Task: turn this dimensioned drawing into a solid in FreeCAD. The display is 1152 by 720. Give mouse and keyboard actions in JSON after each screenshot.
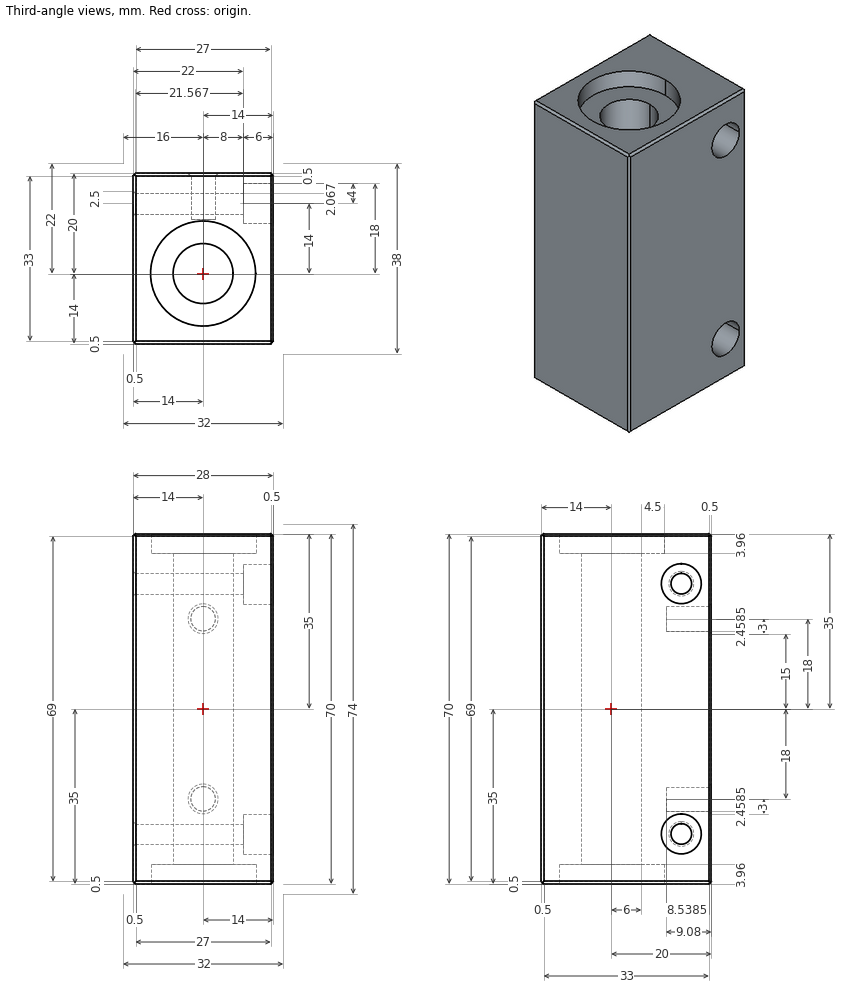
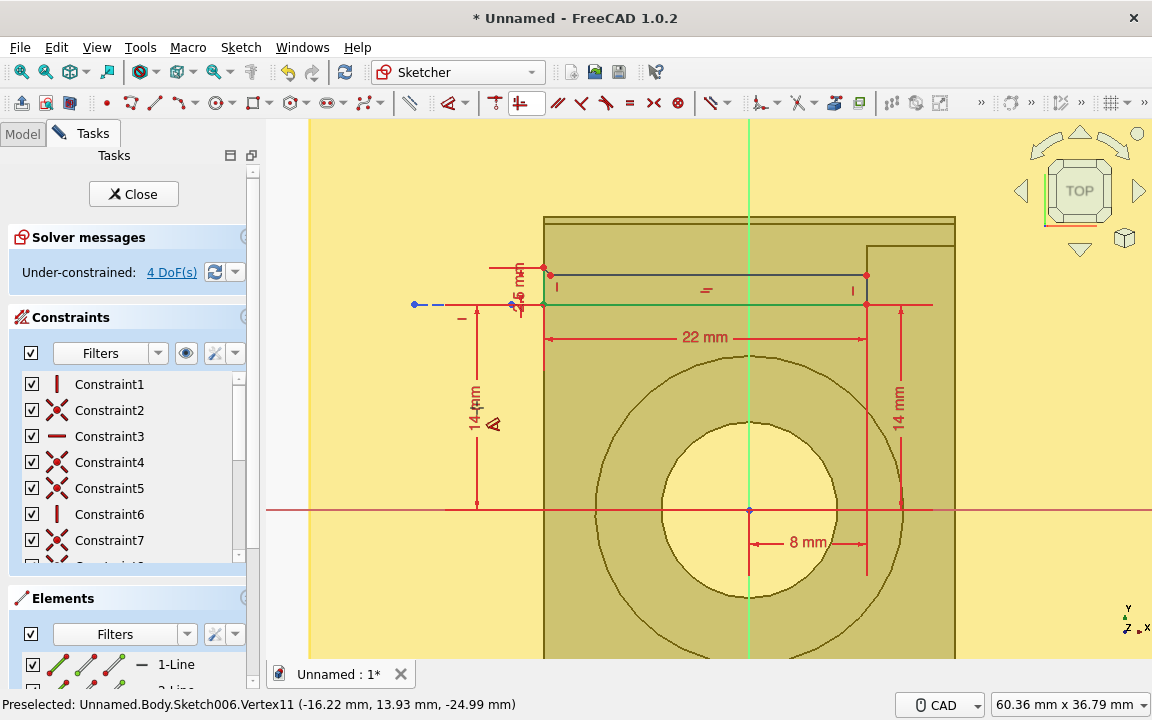
{"action": "scroll", "coordinate": [867, 293], "scroll_direction": "up", "scroll_amount": 2}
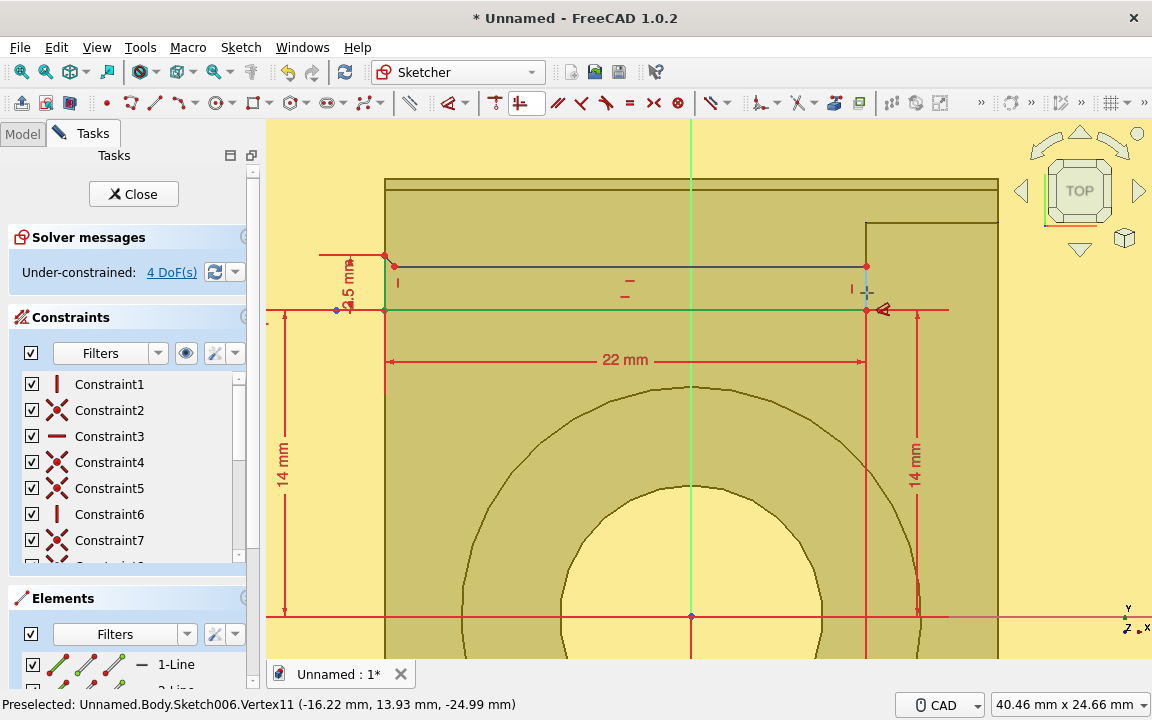
{"action": "left_click", "coordinate": [866, 293]}
{"action": "left_click", "coordinate": [900, 288]}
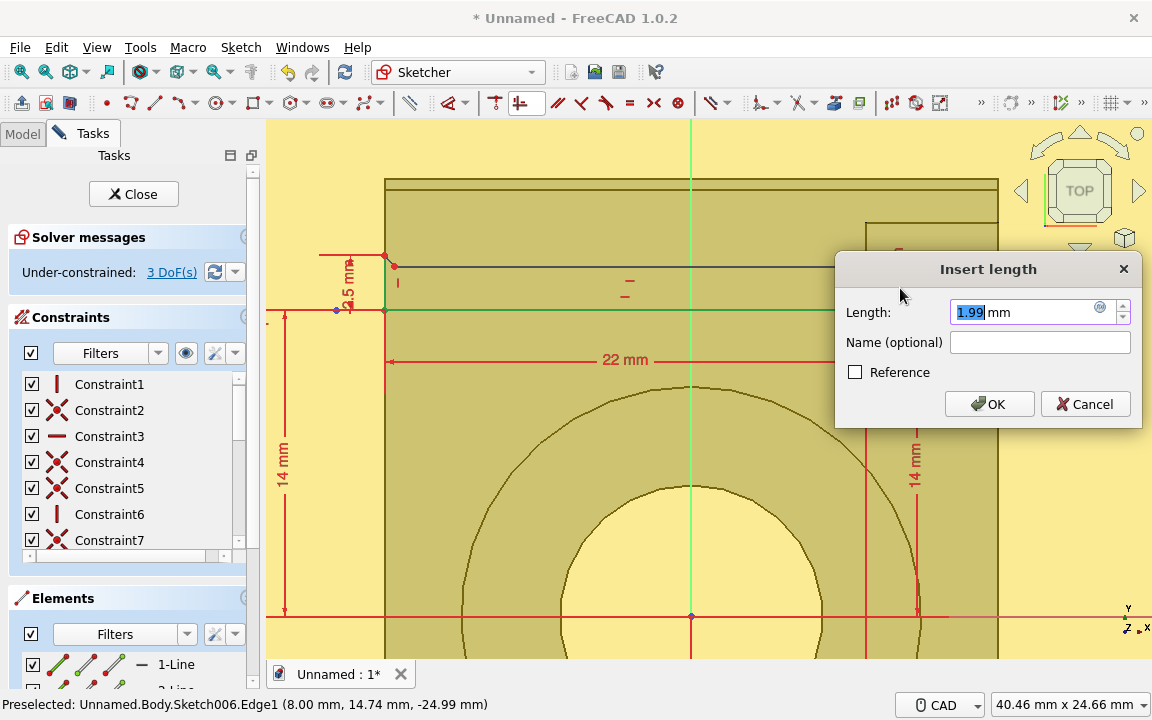
{"action": "type", "text": "2.067"}
{"action": "key", "text": "Return"}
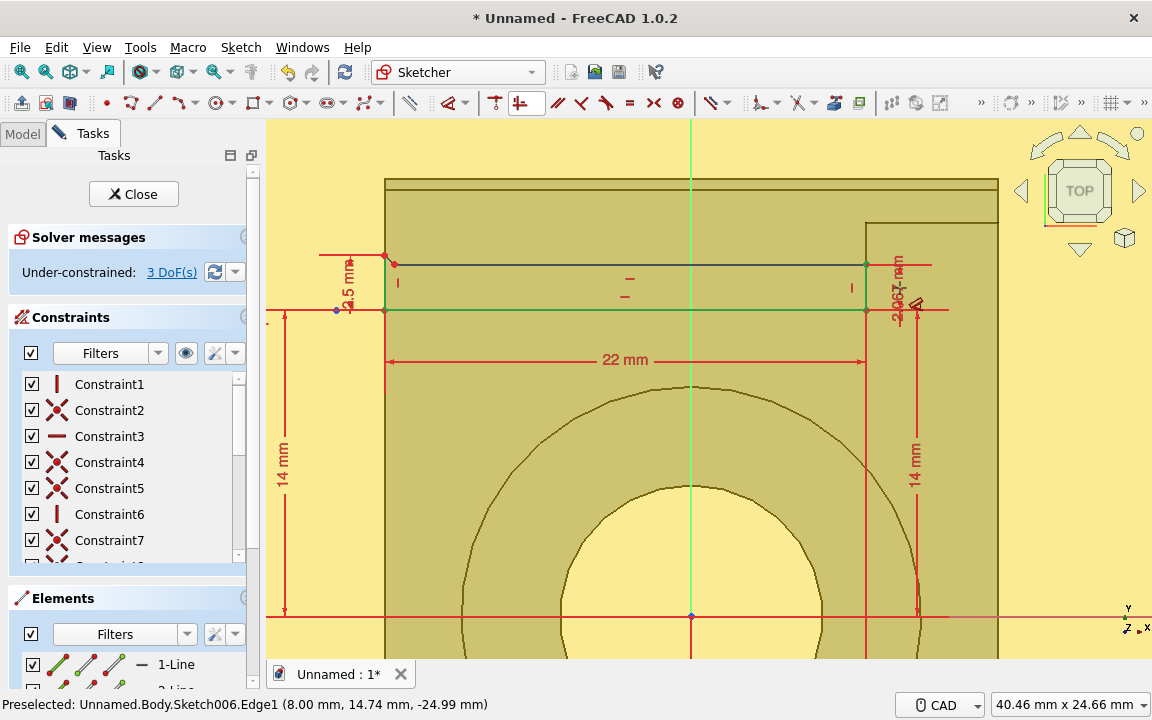
{"action": "left_click", "coordinate": [725, 265]}
{"action": "left_click", "coordinate": [631, 231]}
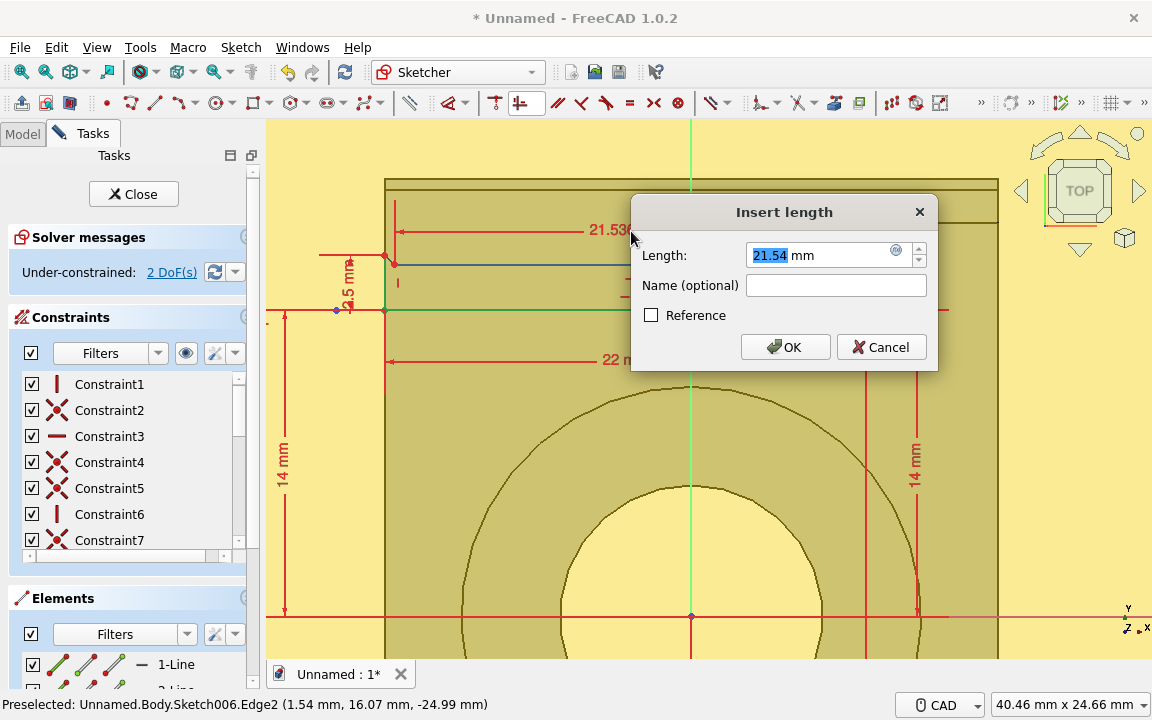
{"action": "type", "text": "21.567"}
{"action": "key", "text": "Return"}
{"action": "key", "text": "Escape"}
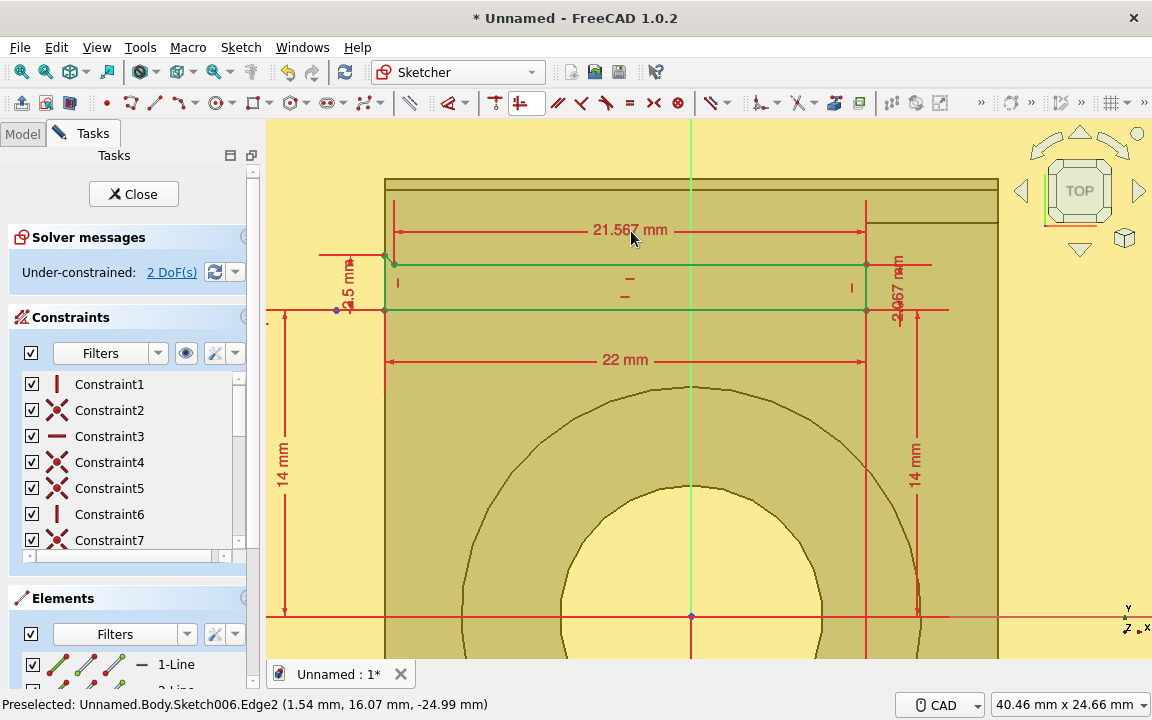
{"action": "left_click", "coordinate": [134, 194]}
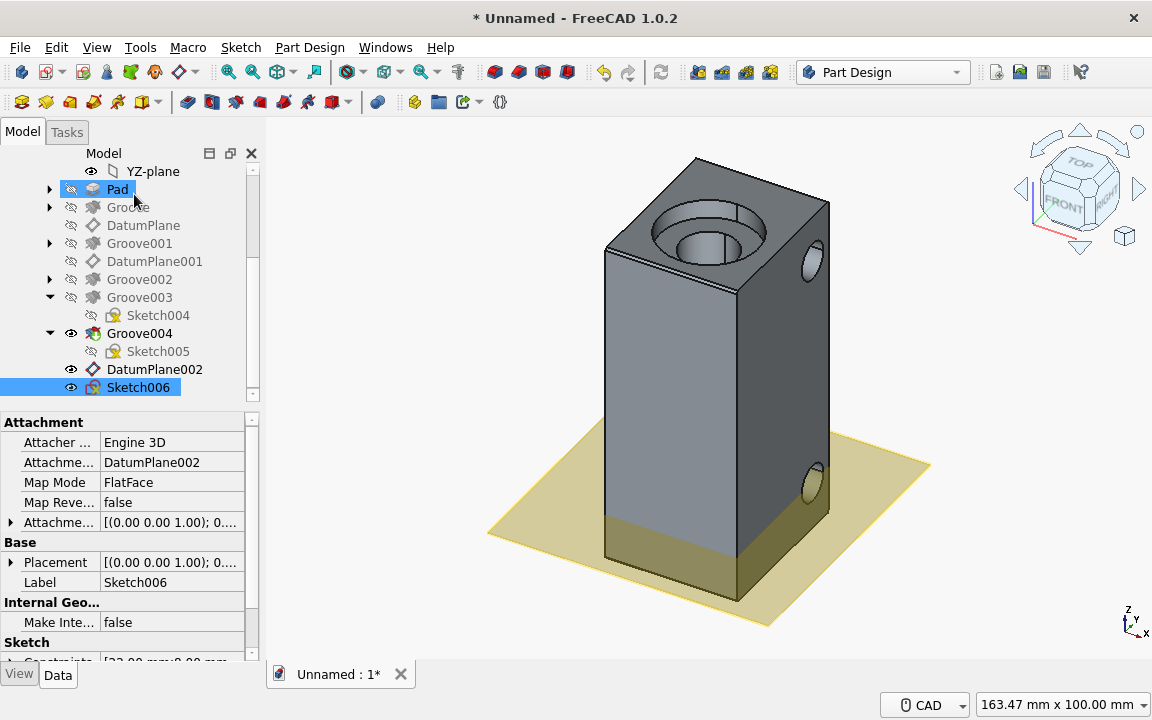
{"action": "left_click", "coordinate": [236, 102]}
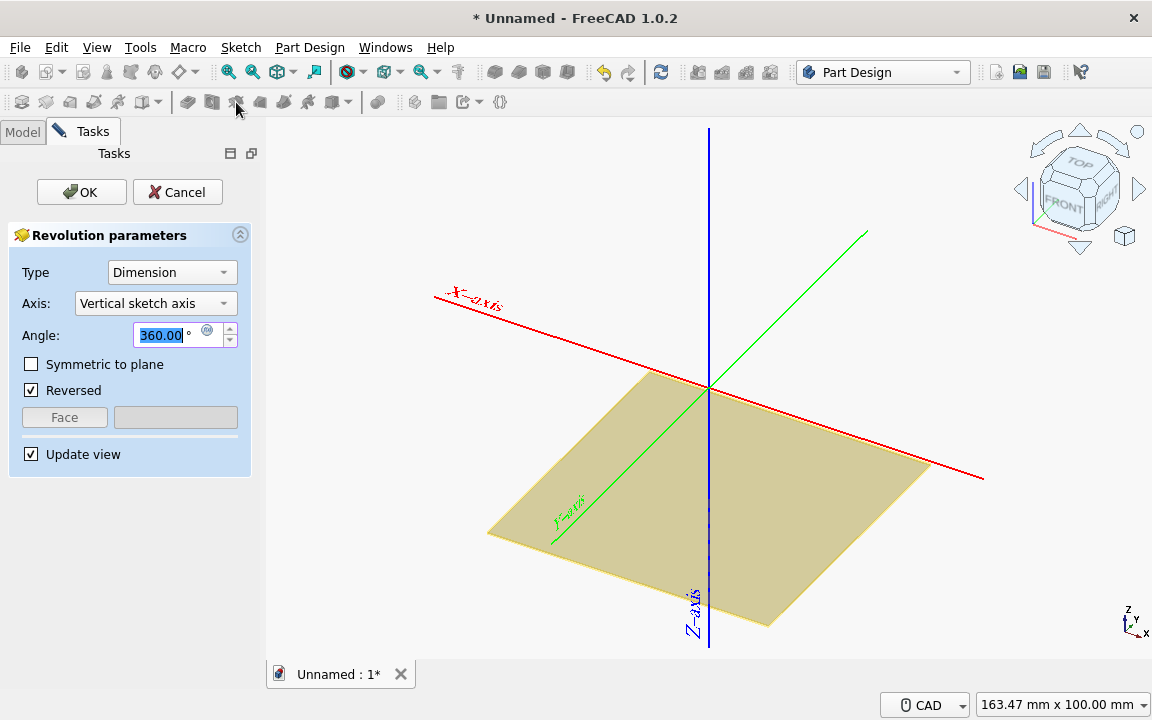
{"action": "left_click", "coordinate": [156, 304]}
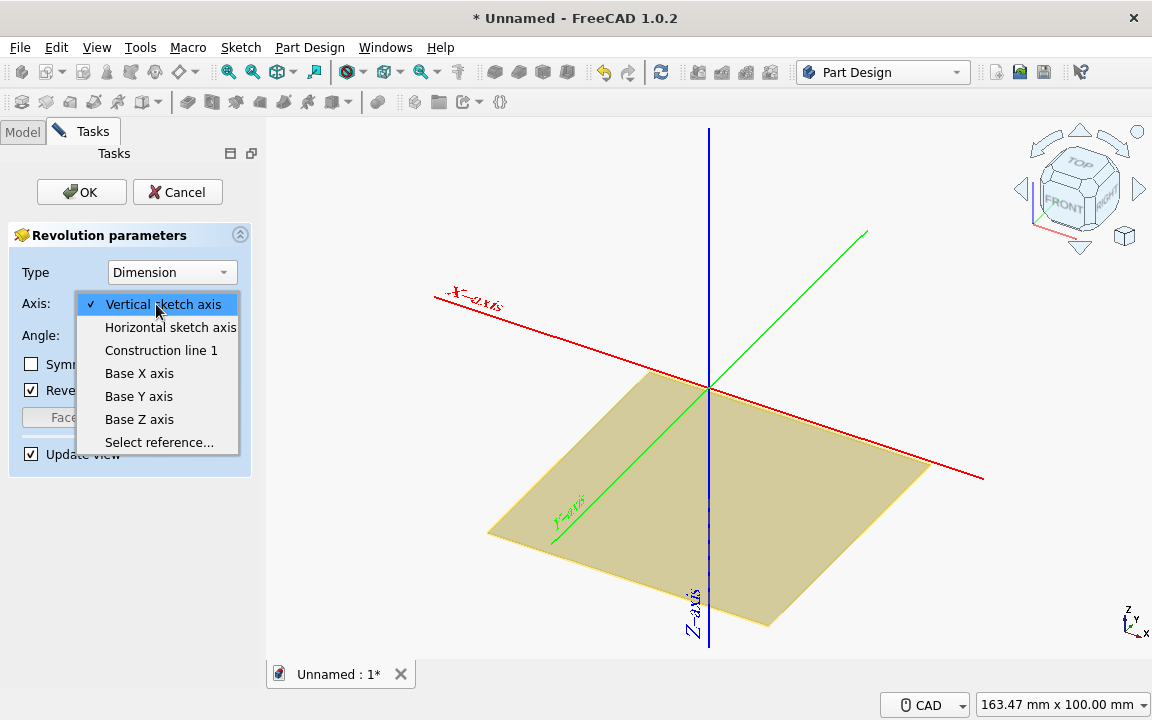
{"action": "left_click", "coordinate": [156, 350]}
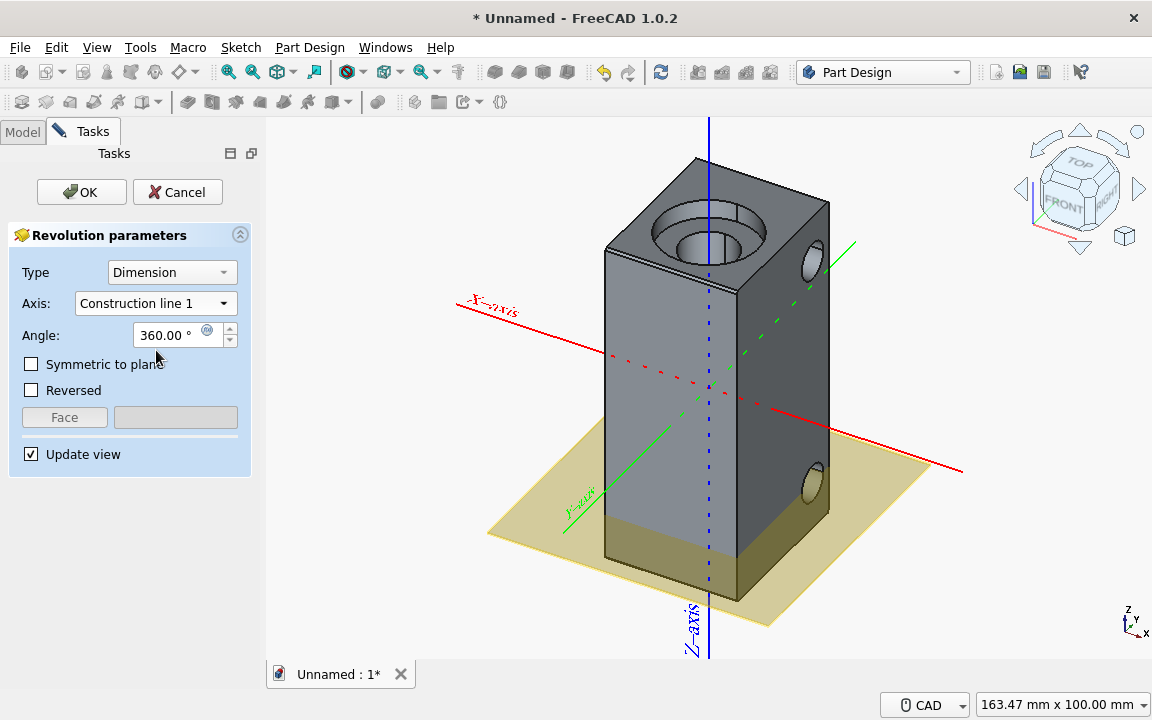
{"action": "left_click", "coordinate": [82, 192]}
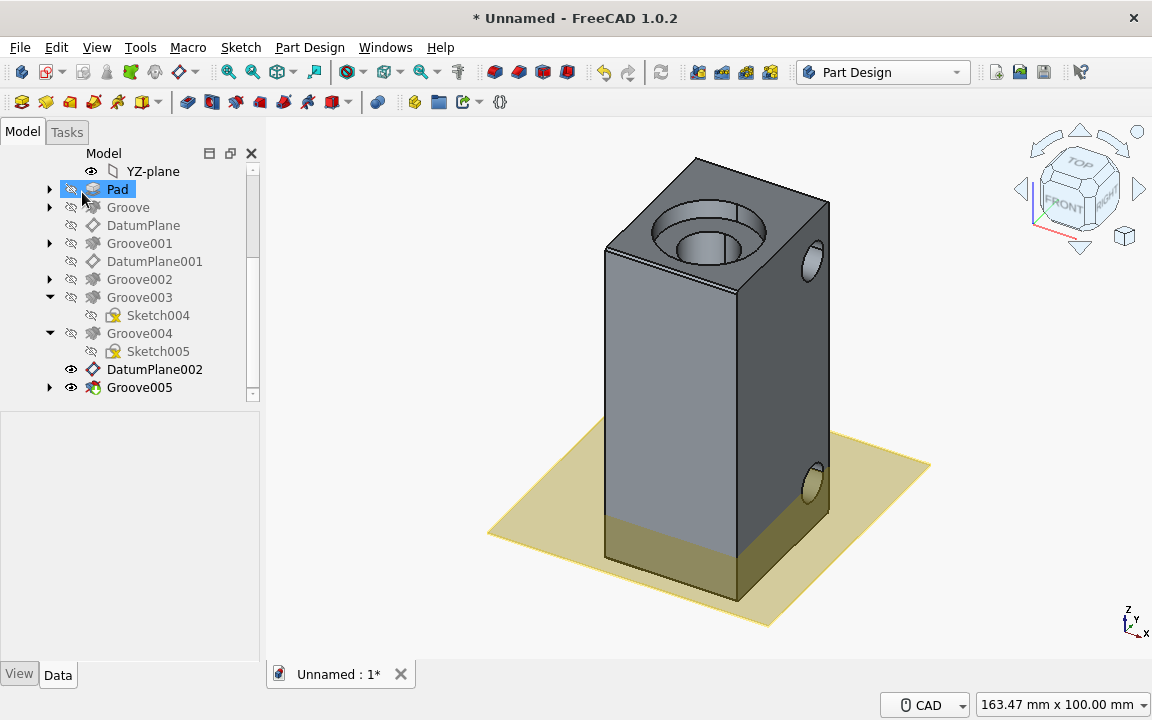
{"action": "left_click", "coordinate": [116, 369]}
{"action": "key", "text": "space"}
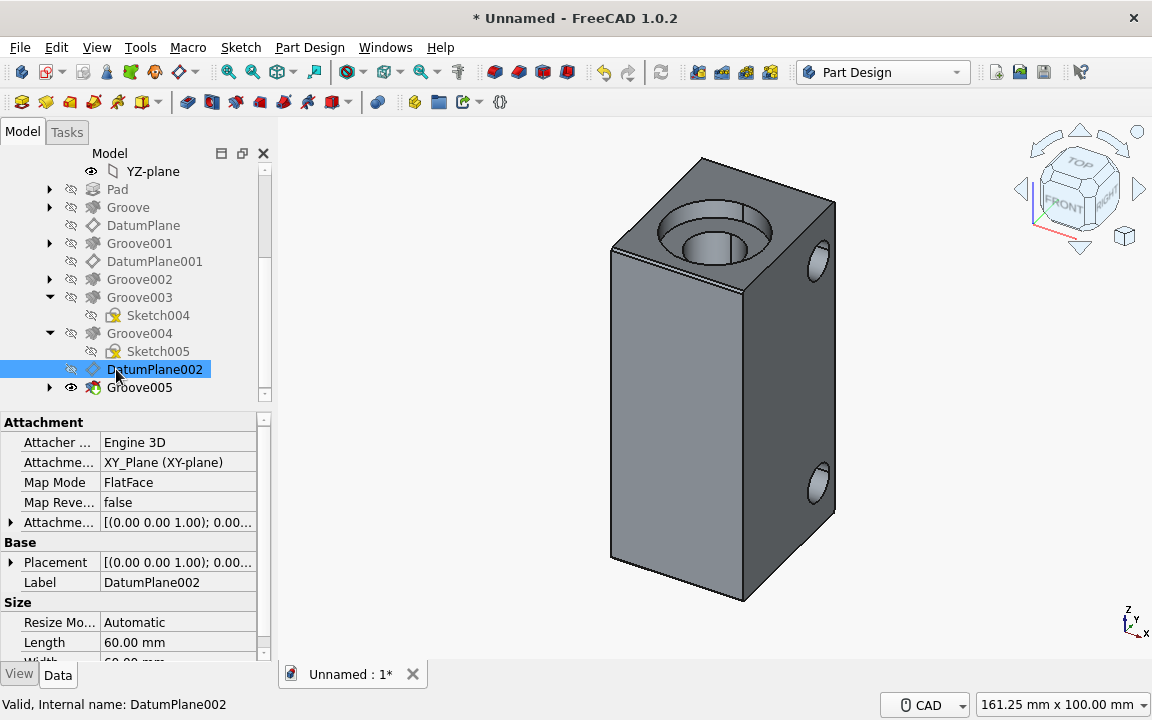
{"action": "scroll", "coordinate": [160, 275], "scroll_direction": "down", "scroll_amount": 3}